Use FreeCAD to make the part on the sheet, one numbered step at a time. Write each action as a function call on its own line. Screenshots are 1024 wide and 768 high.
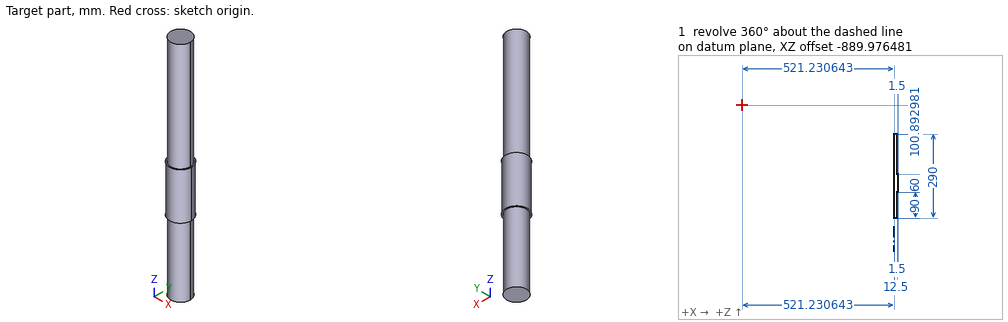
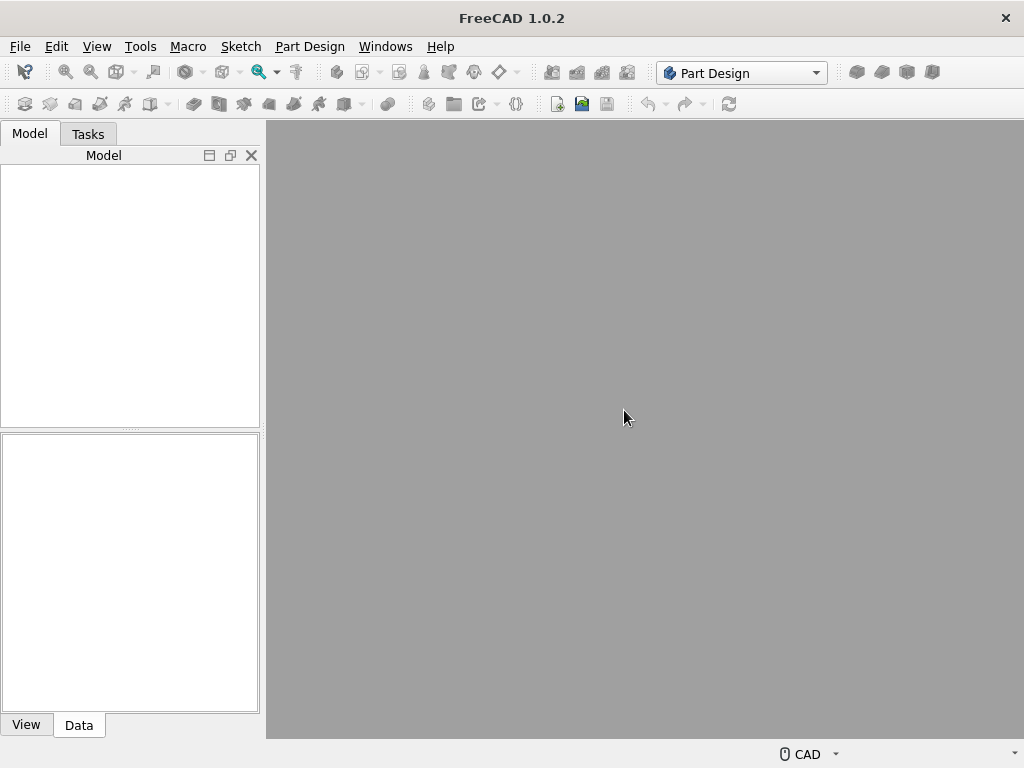
click(557, 104)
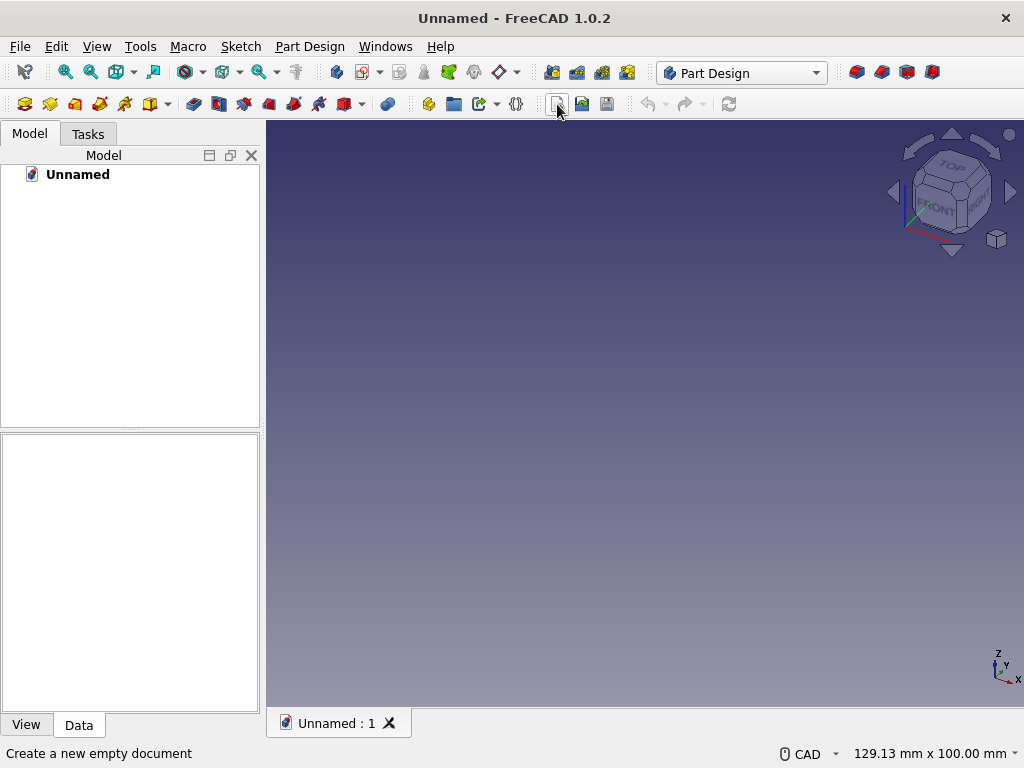
click(337, 72)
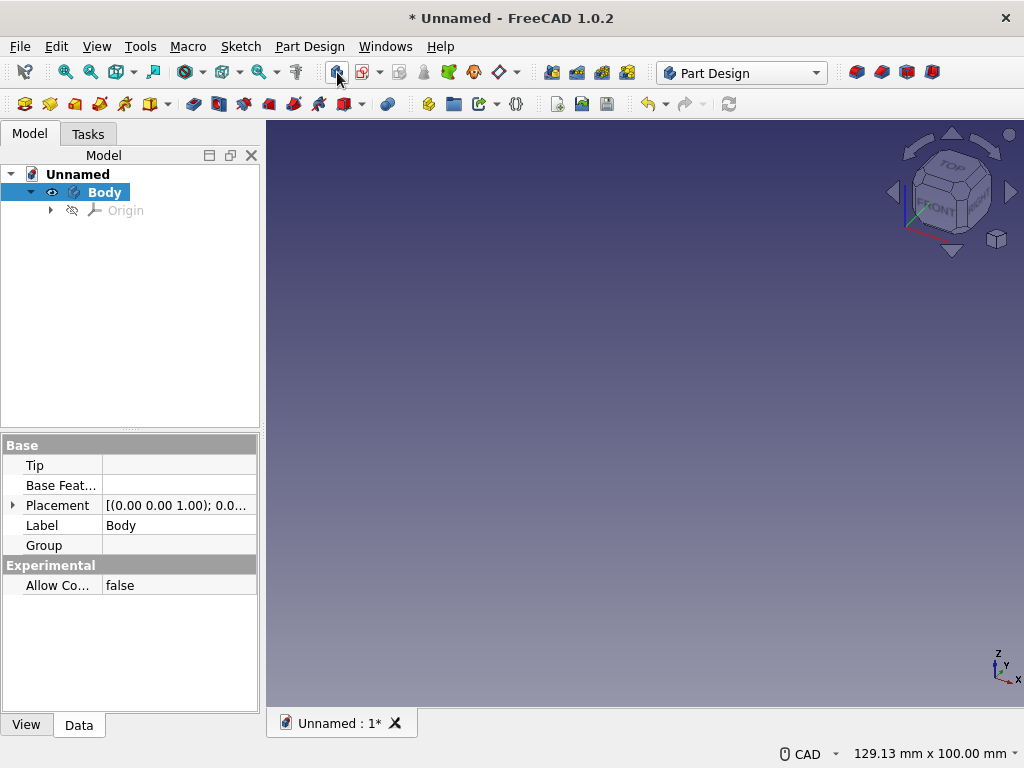
click(51, 210)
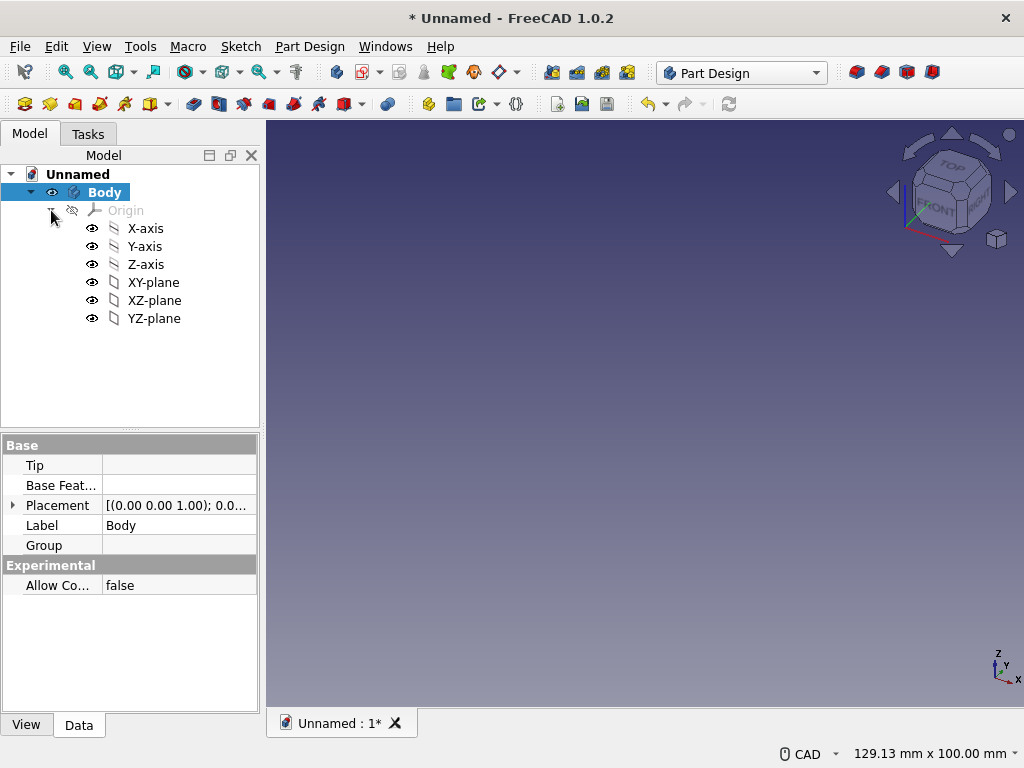
click(137, 300)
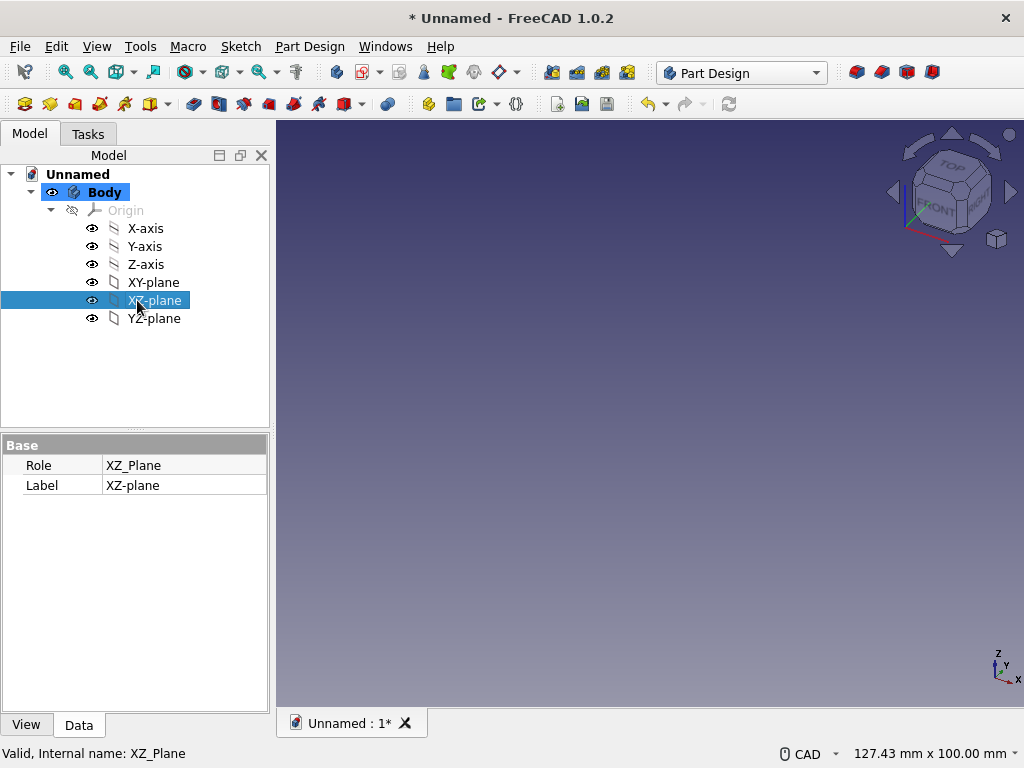
click(498, 72)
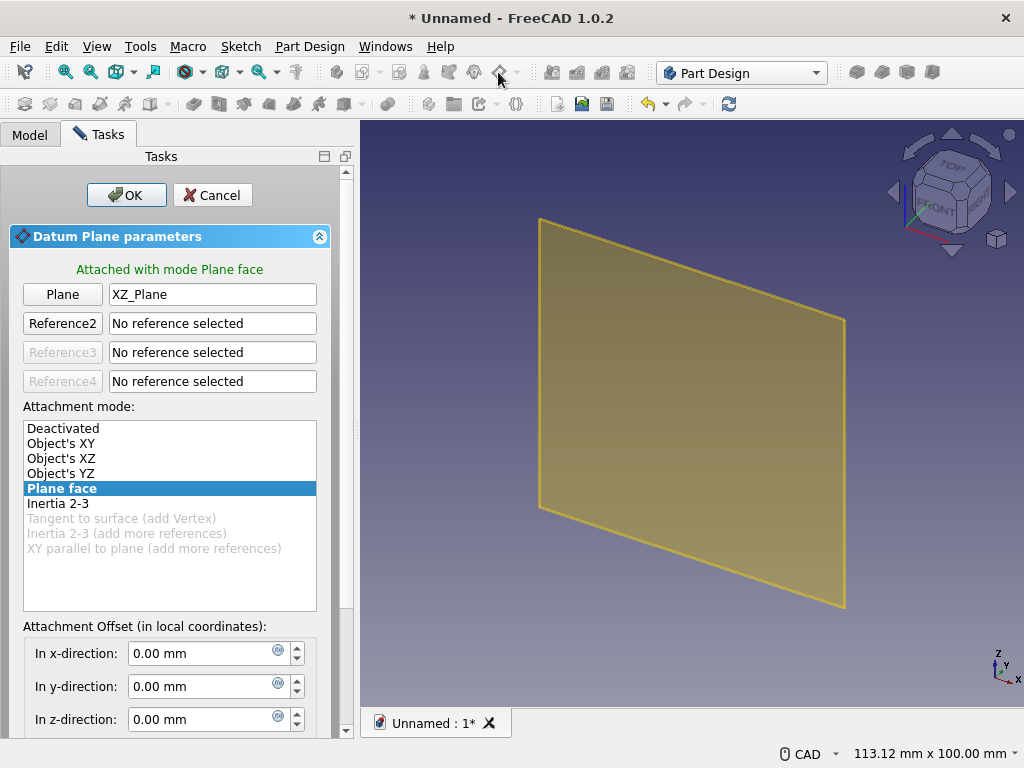
triple_click(210, 720)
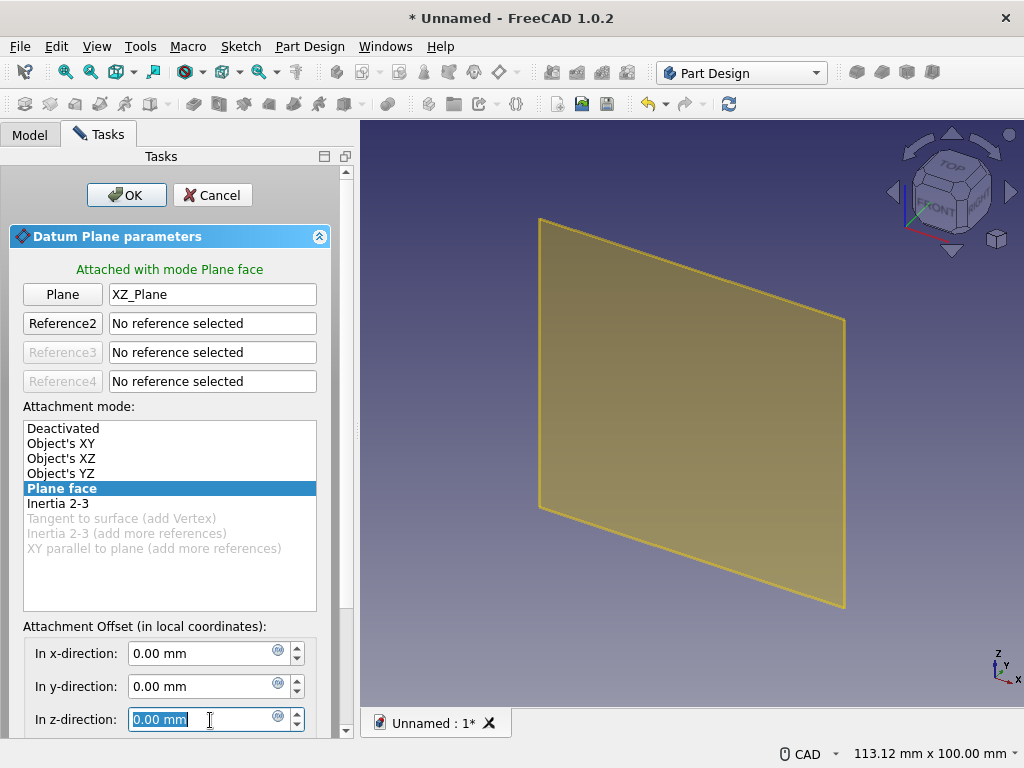
text(-889.976481)
key(Tab)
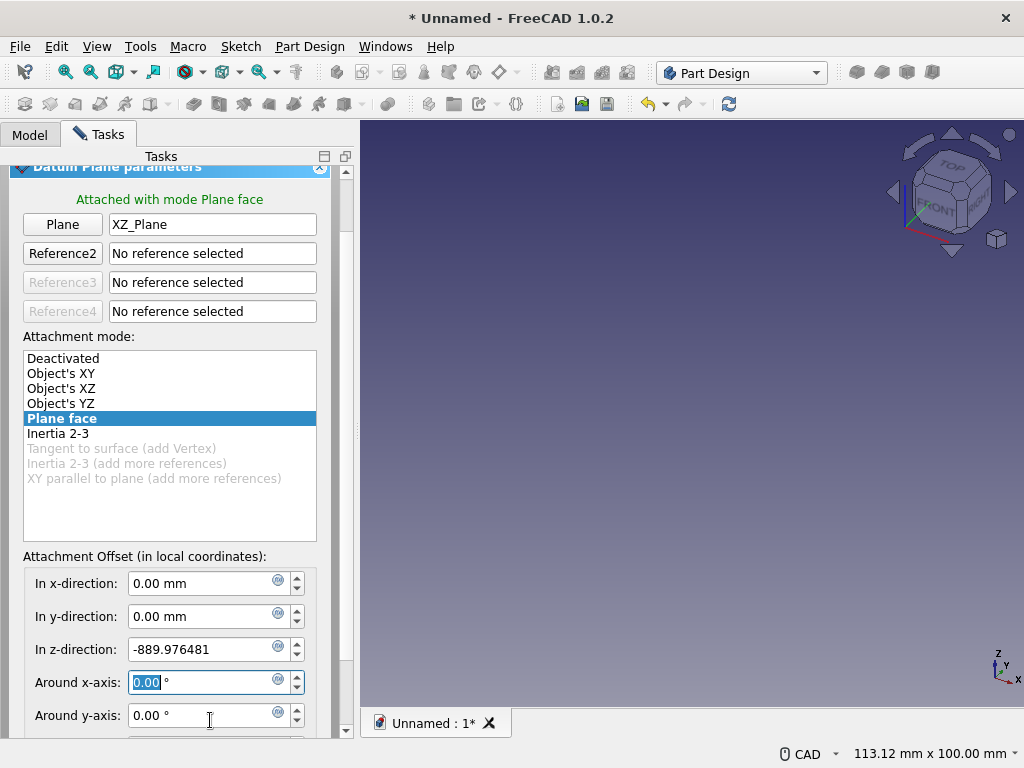
scroll(346, 452, up, 2)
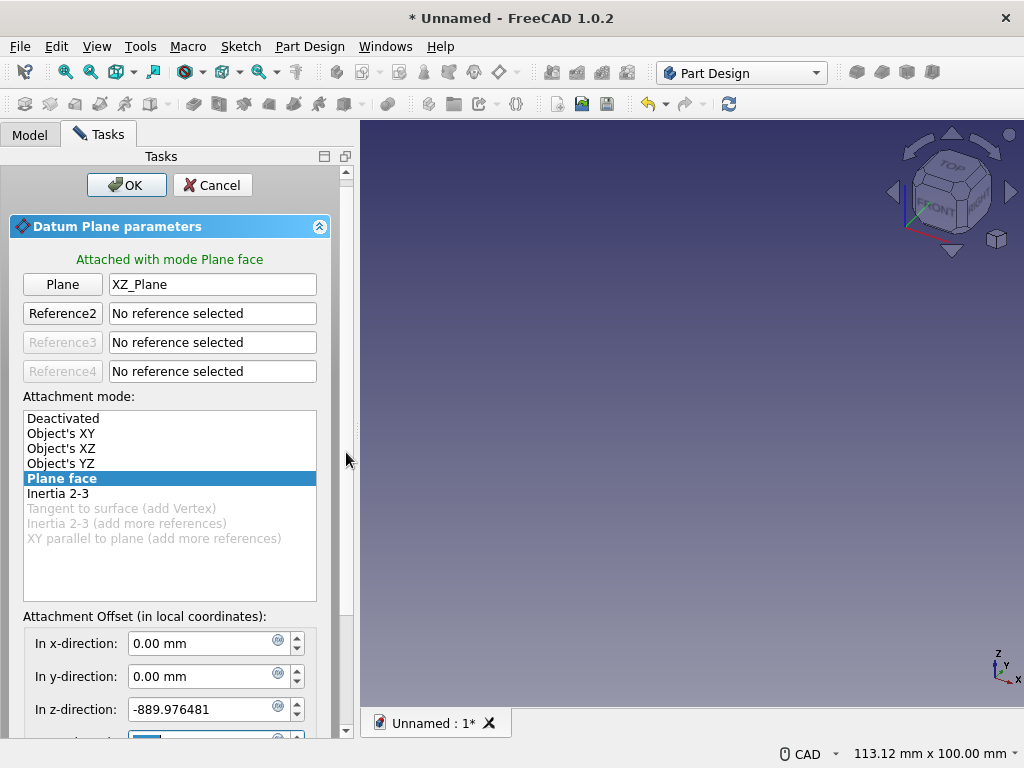
click(127, 195)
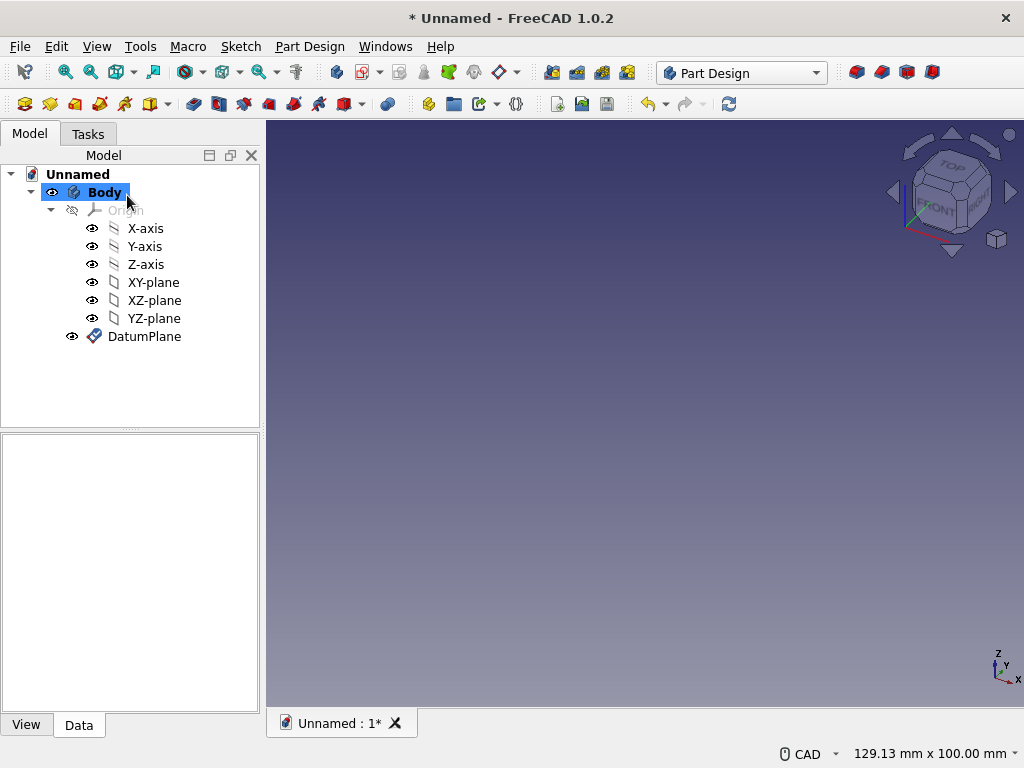
click(117, 336)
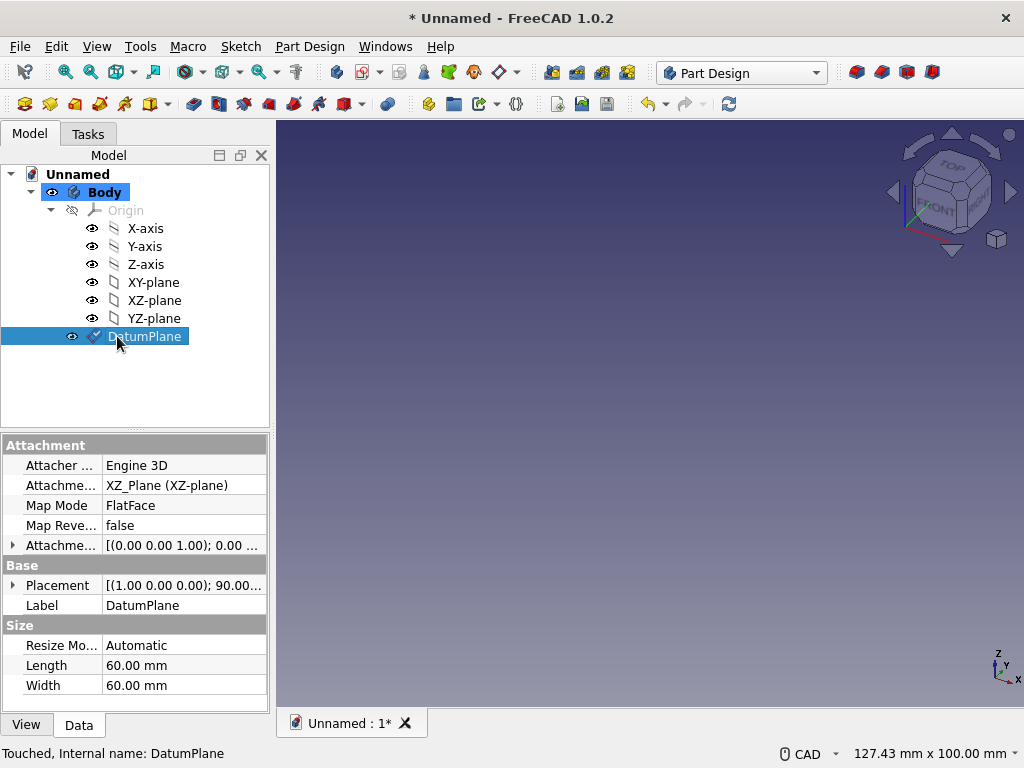
click(362, 72)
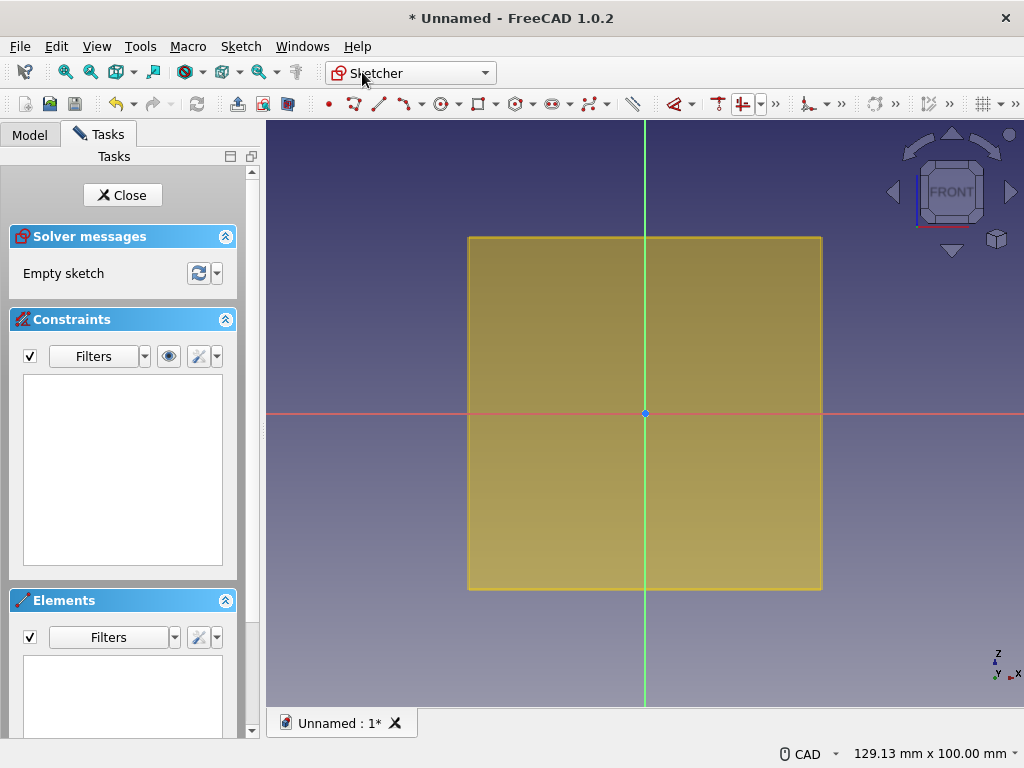
scroll(320, 181, down, 10)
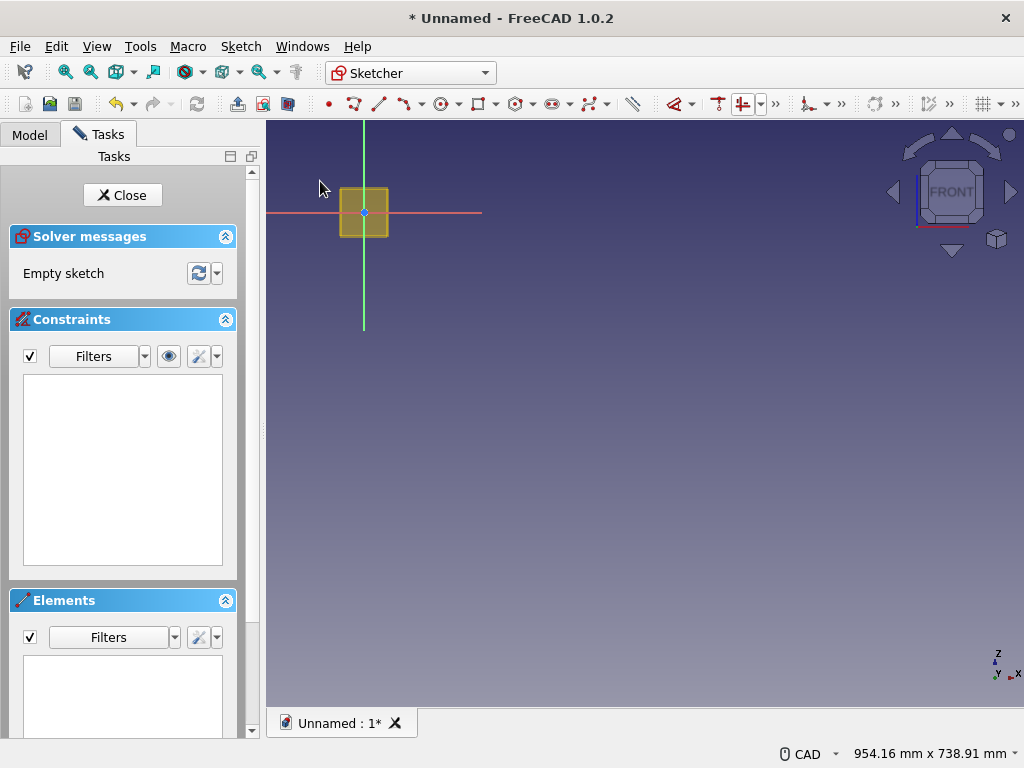
click(354, 104)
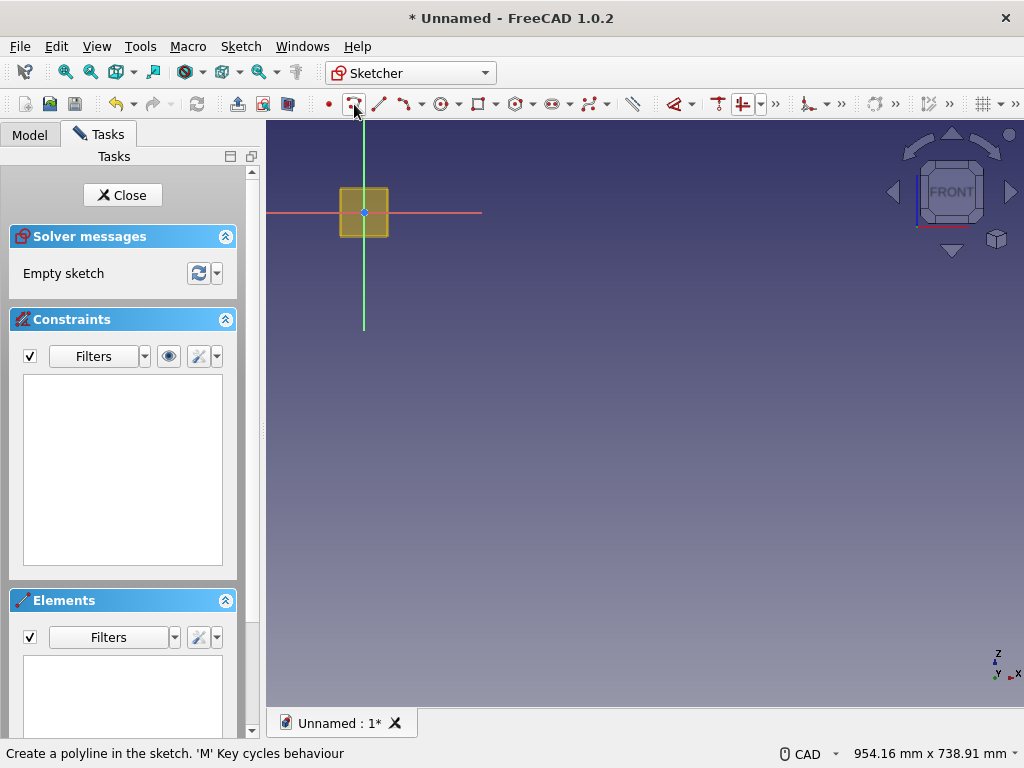
click(778, 293)
click(778, 523)